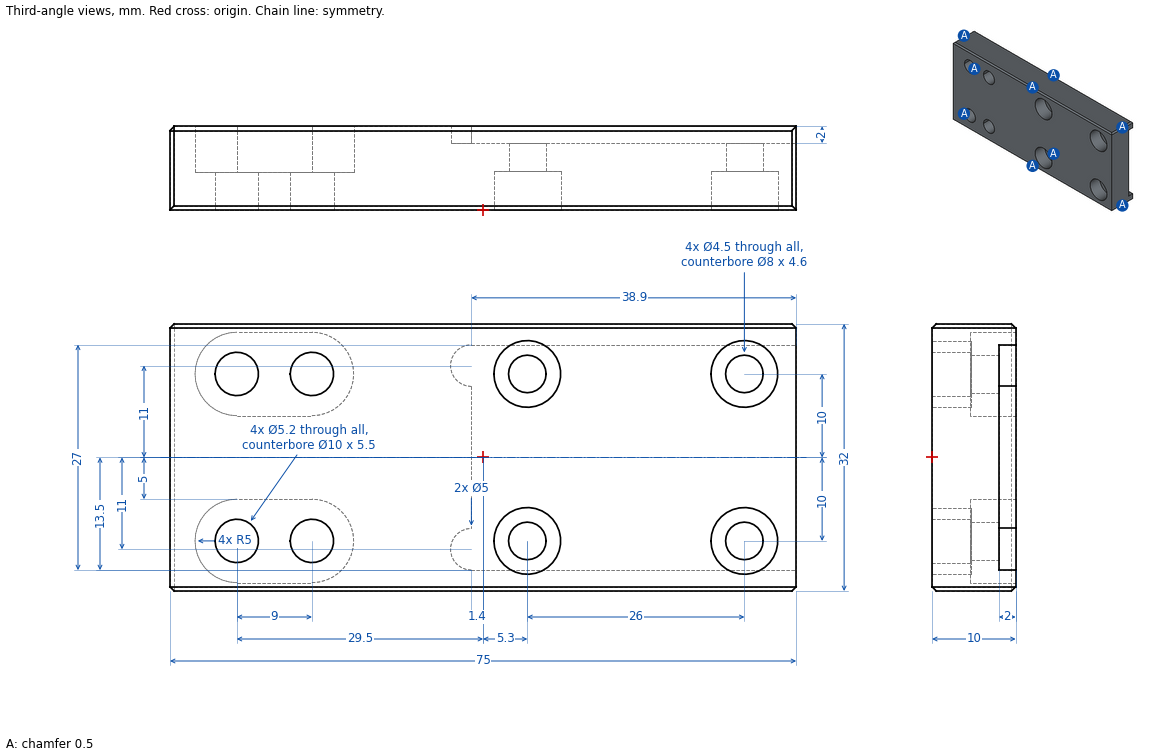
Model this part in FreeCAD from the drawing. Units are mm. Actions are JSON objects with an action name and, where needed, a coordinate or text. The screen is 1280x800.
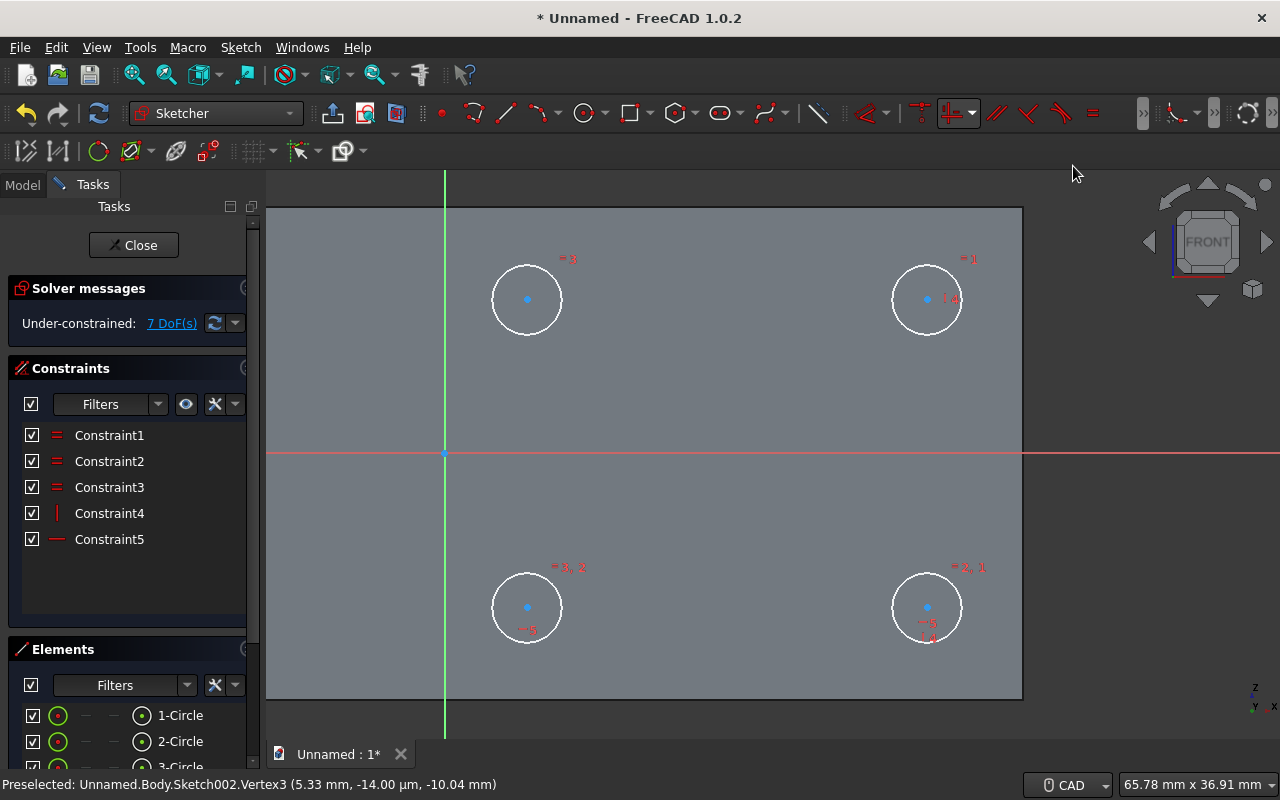
{"action": "left_click", "coordinate": [527, 608]}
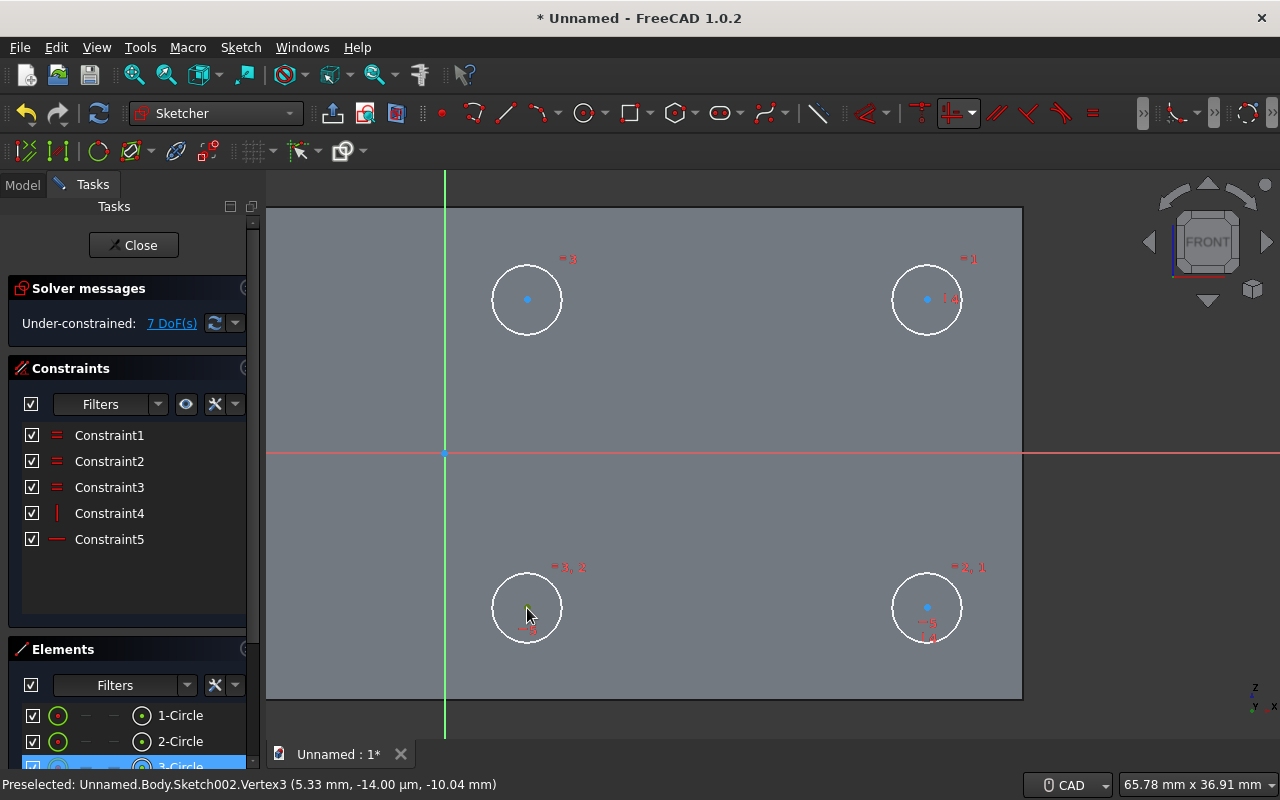
{"action": "left_click", "coordinate": [527, 300]}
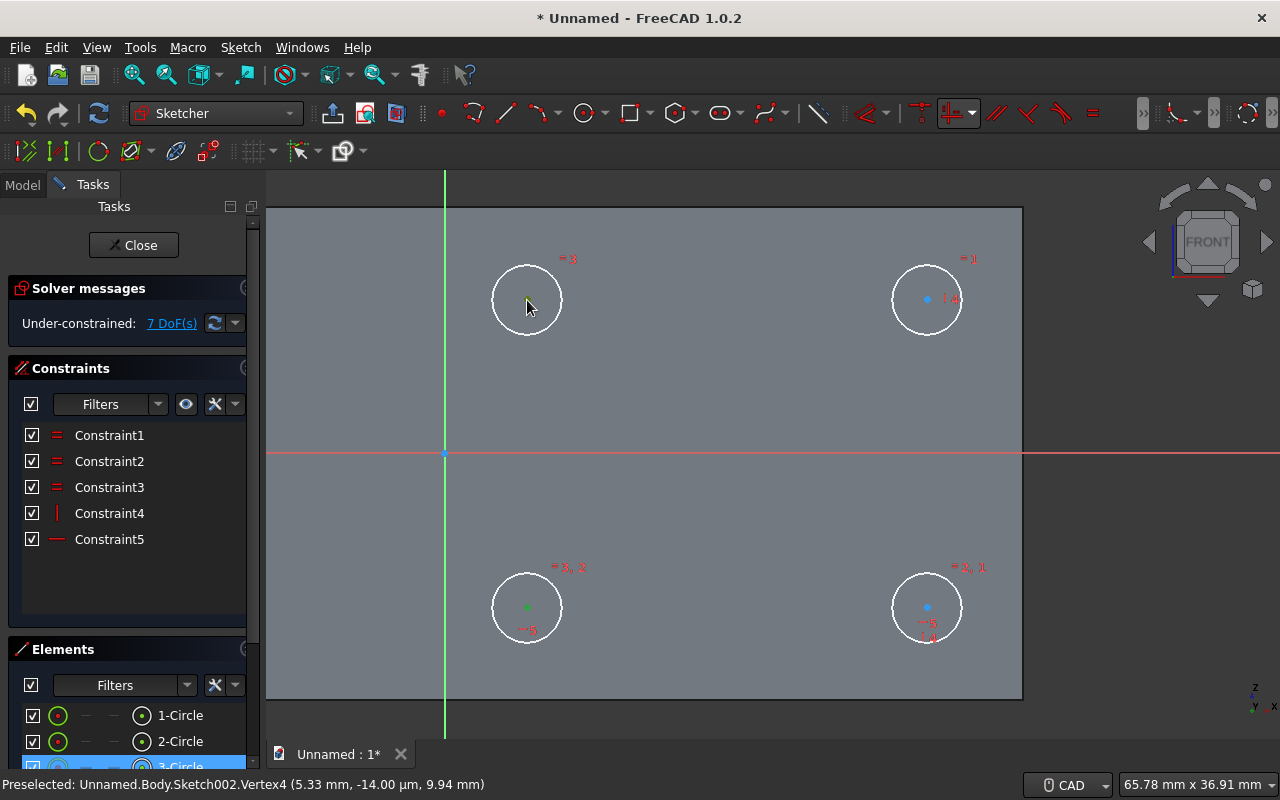
{"action": "left_click", "coordinate": [974, 114]}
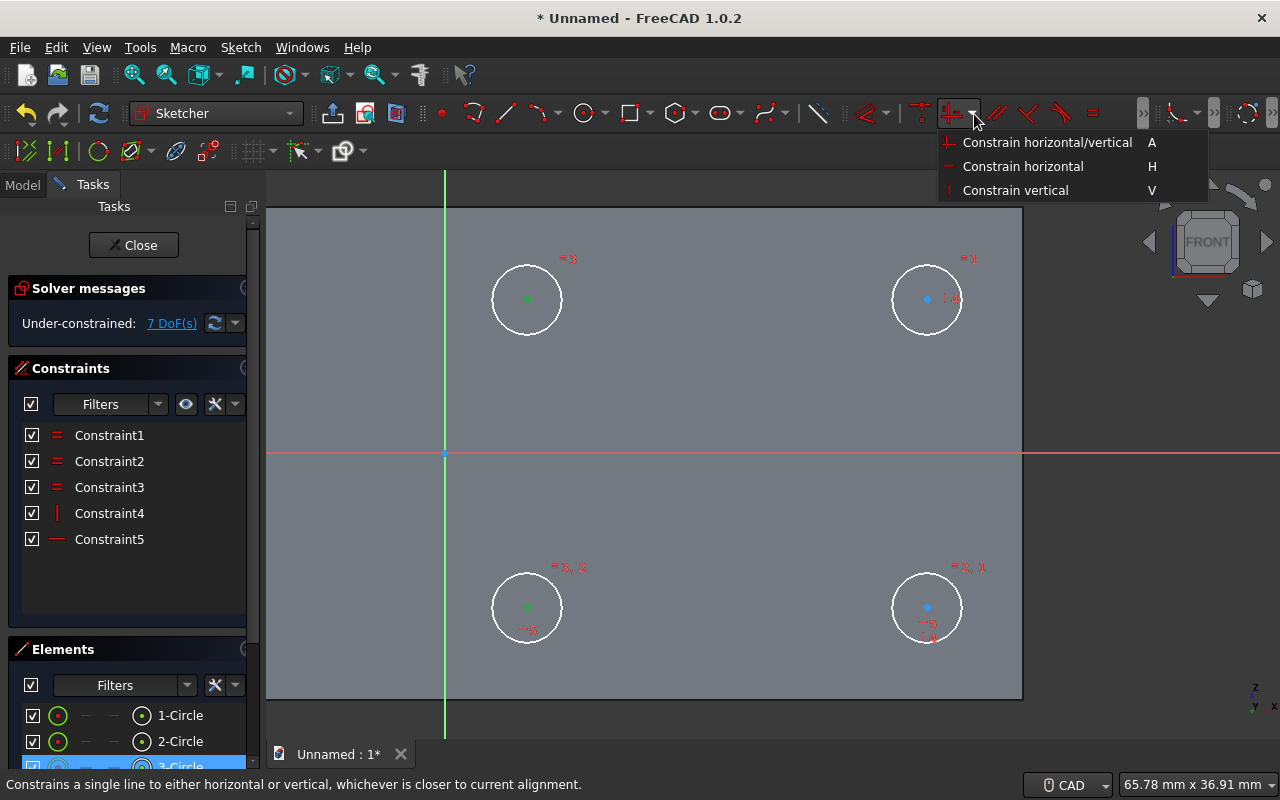
{"action": "left_click", "coordinate": [1073, 190]}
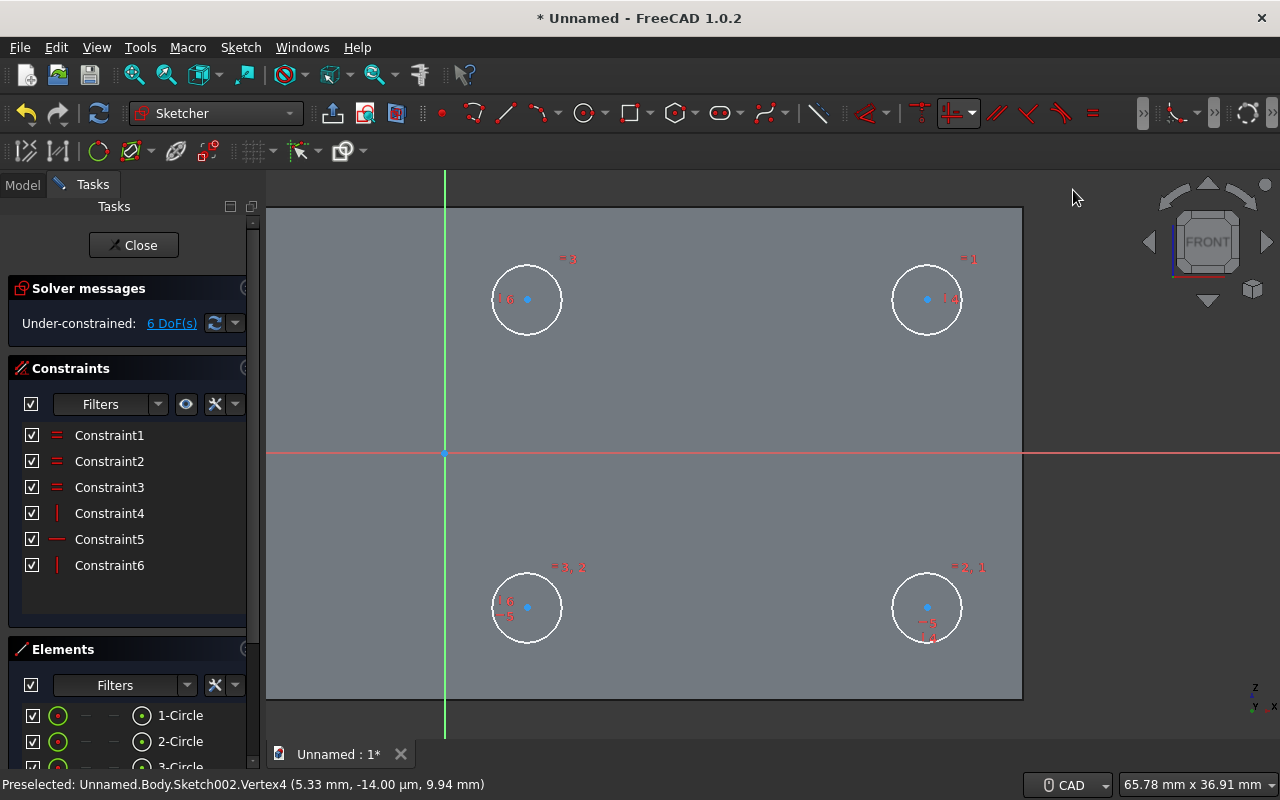
{"action": "left_click", "coordinate": [927, 300]}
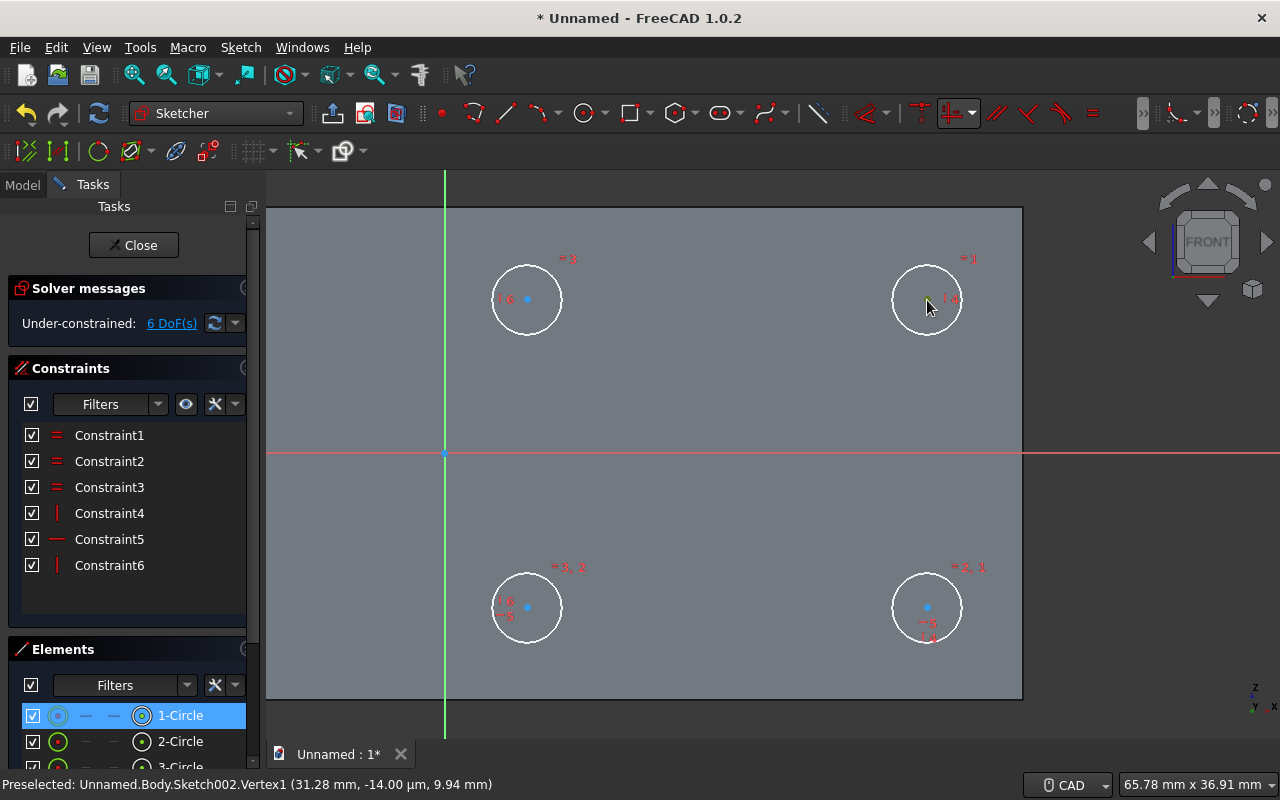
{"action": "left_click", "coordinate": [527, 300]}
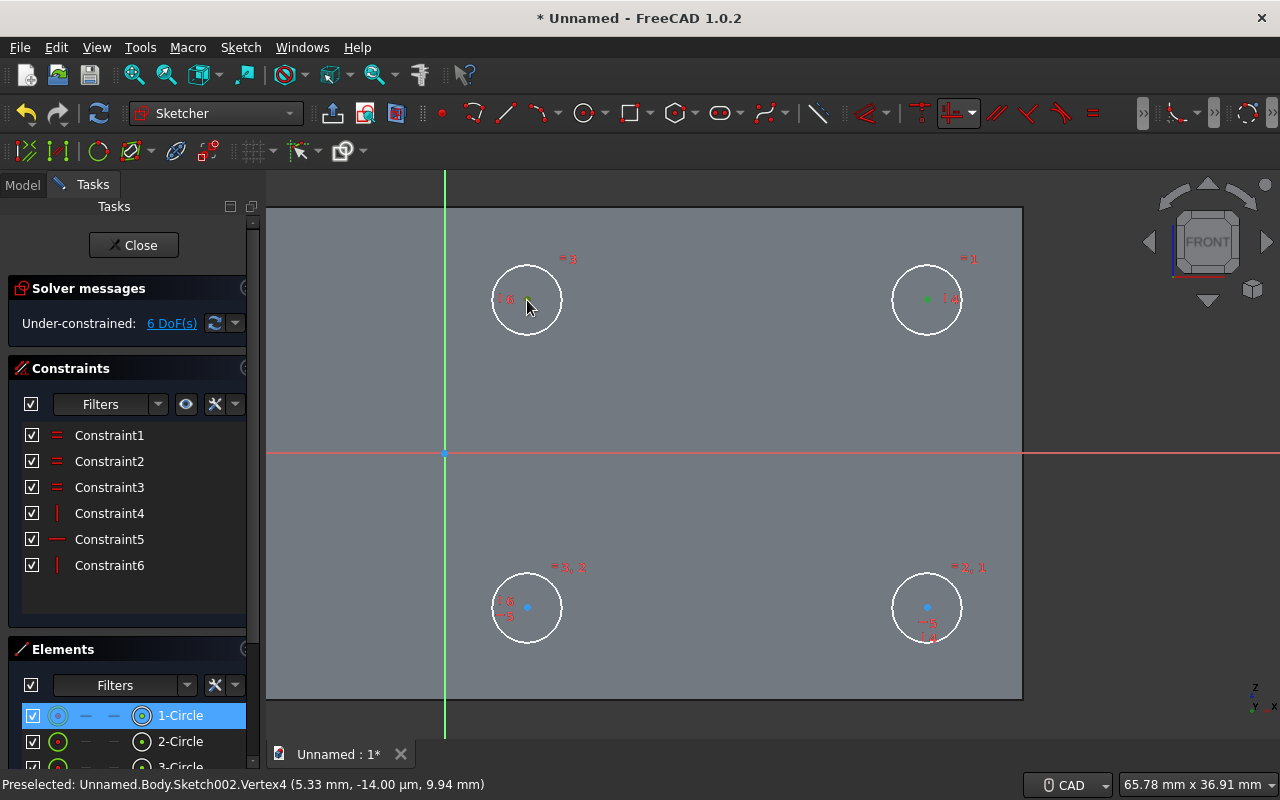
{"action": "left_click", "coordinate": [974, 114]}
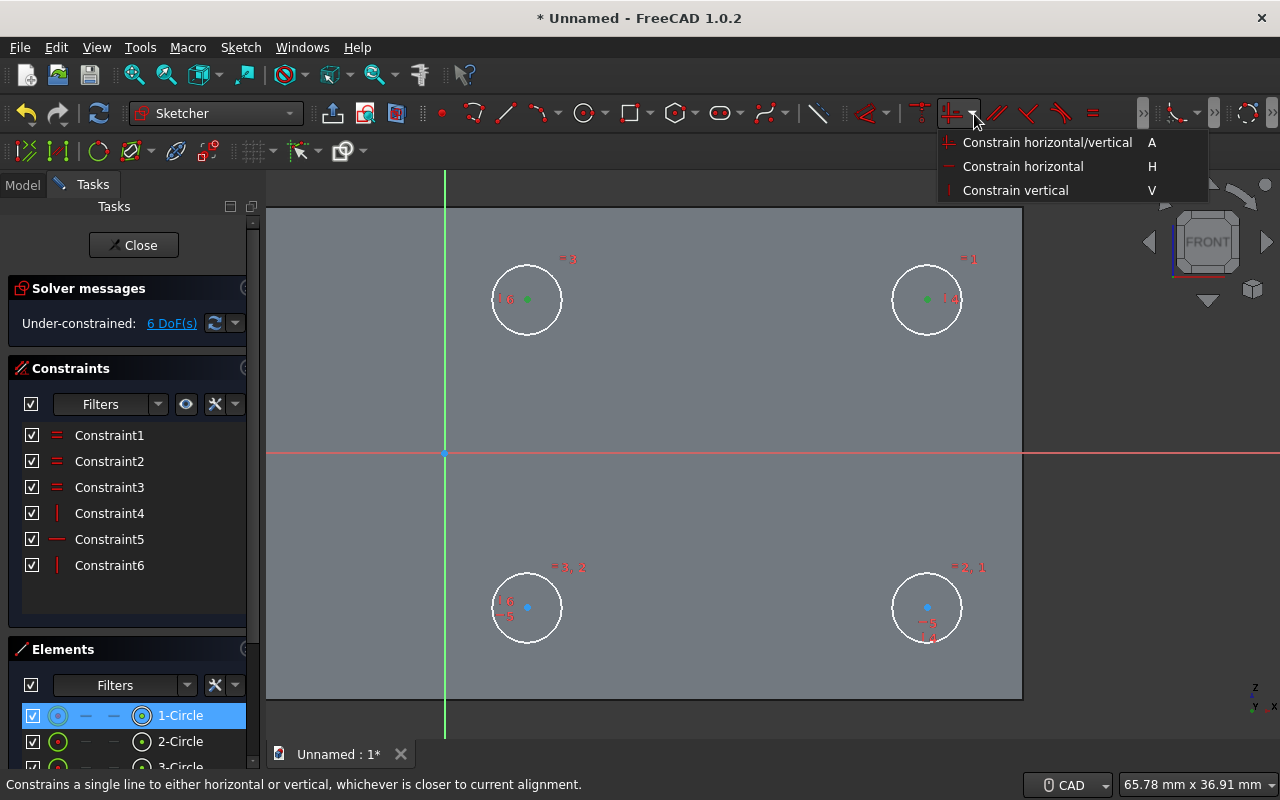
{"action": "left_click", "coordinate": [1073, 166]}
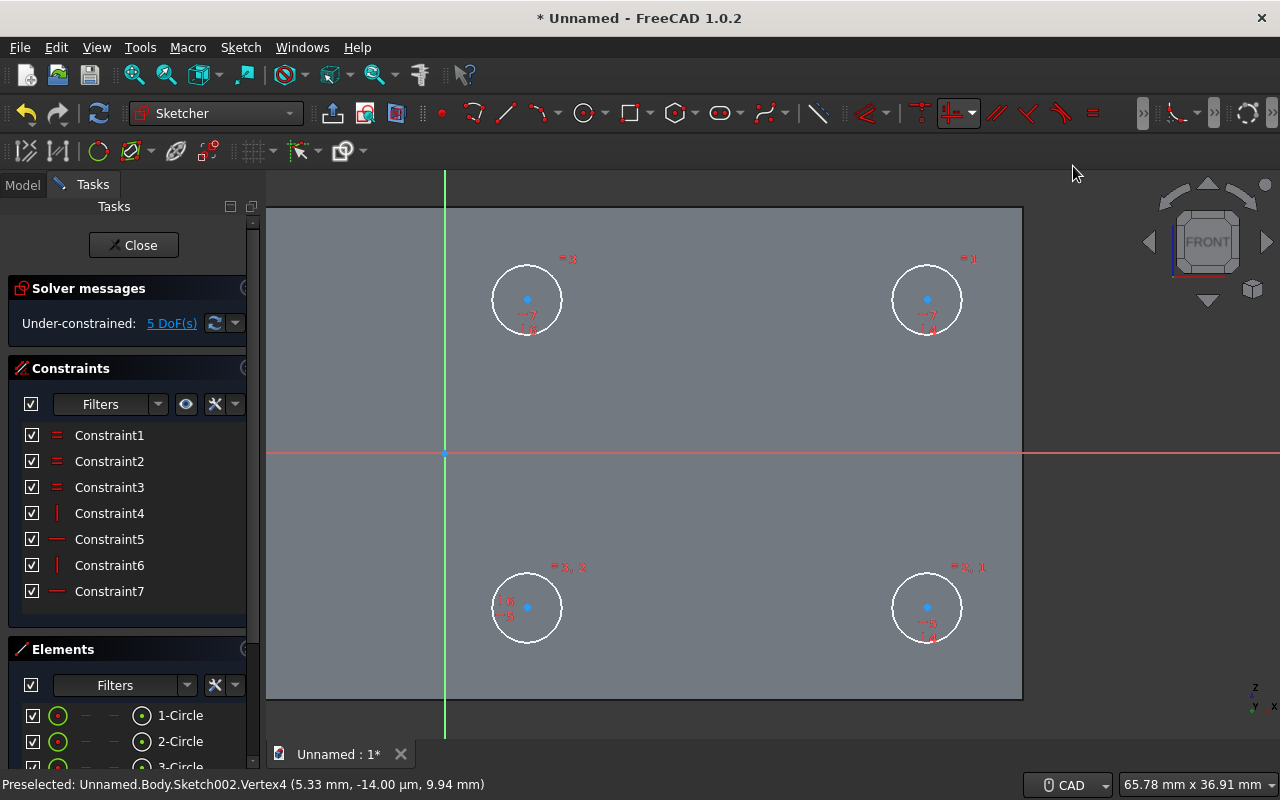
{"action": "left_click", "coordinate": [866, 114]}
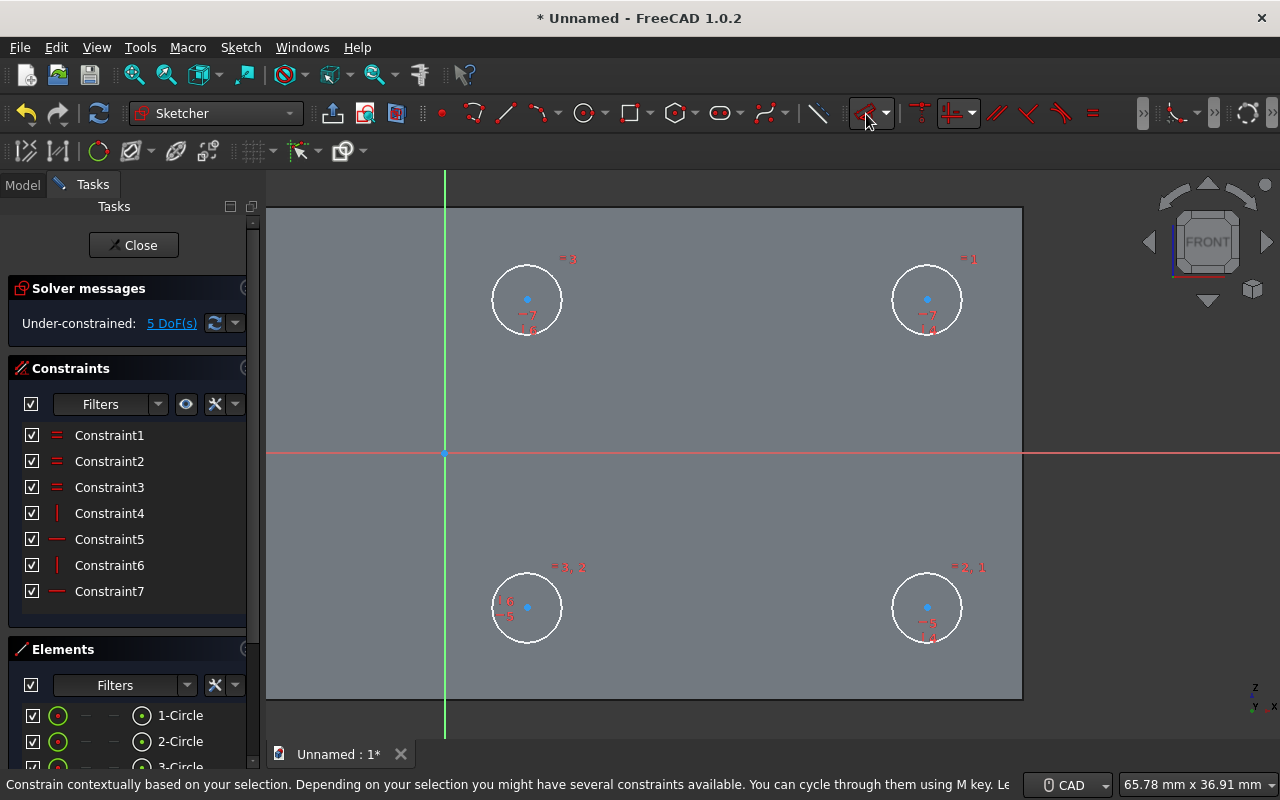
{"action": "left_click", "coordinate": [951, 275]}
{"action": "left_click", "coordinate": [973, 252]}